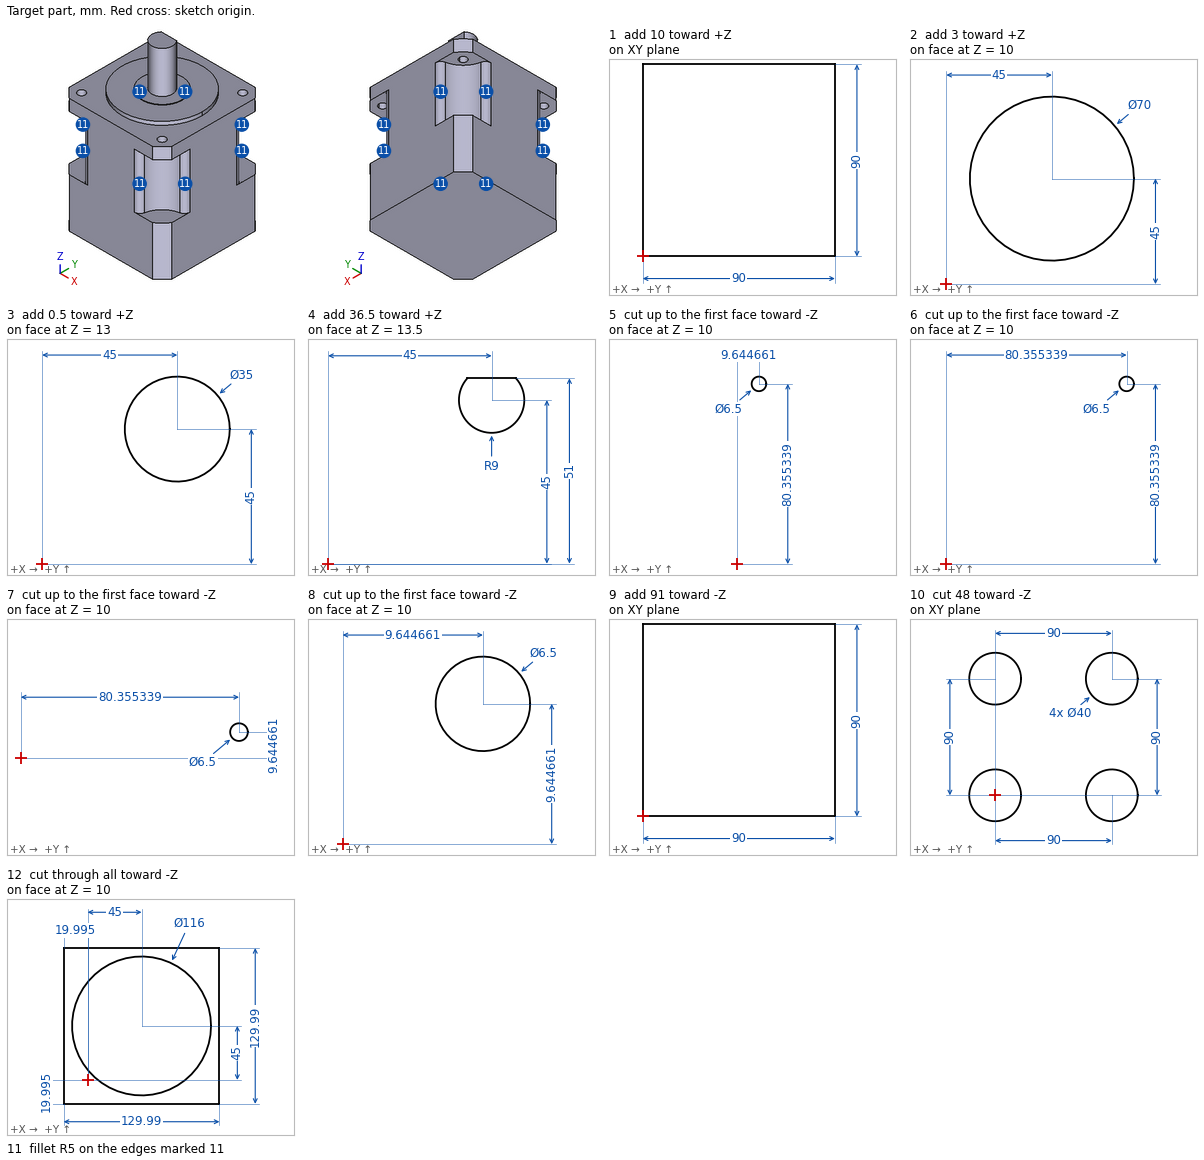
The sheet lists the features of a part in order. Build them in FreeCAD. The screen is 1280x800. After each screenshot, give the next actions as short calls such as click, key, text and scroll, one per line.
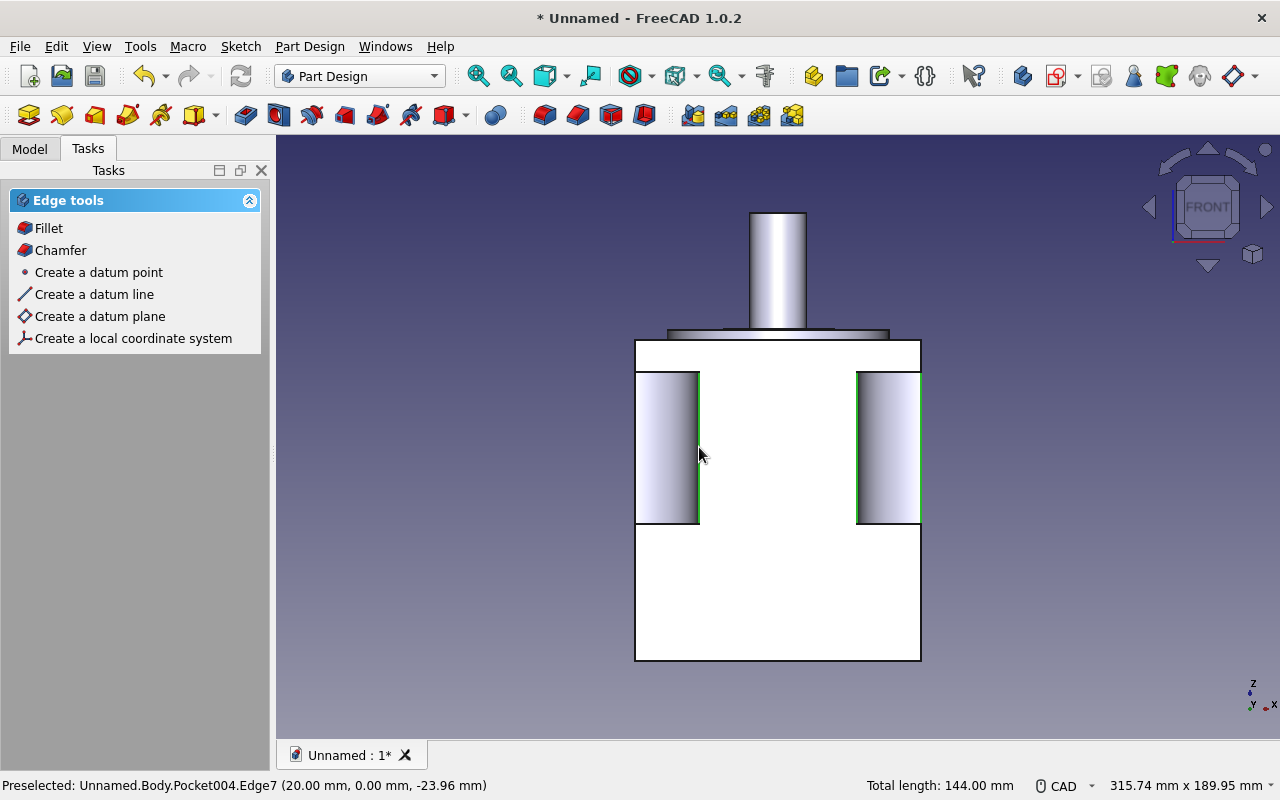
key(3)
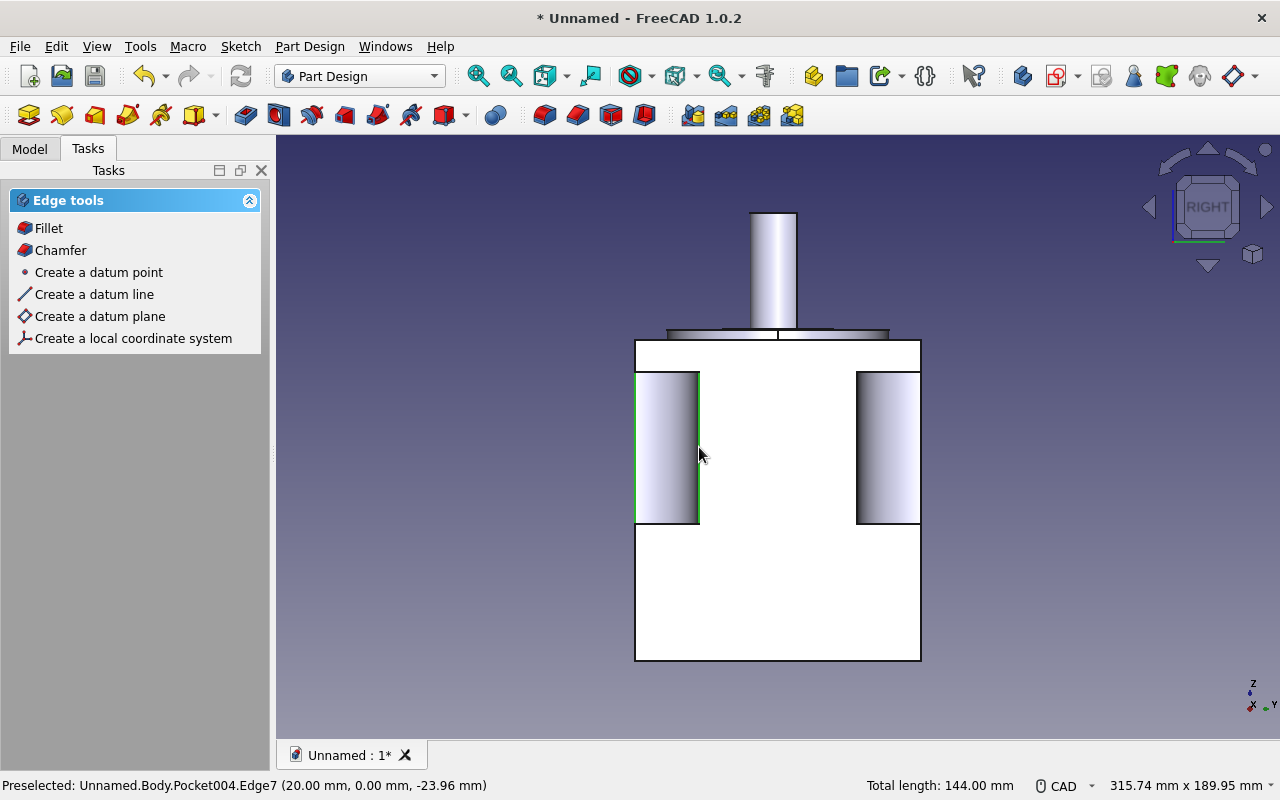
click(857, 447, ctrl)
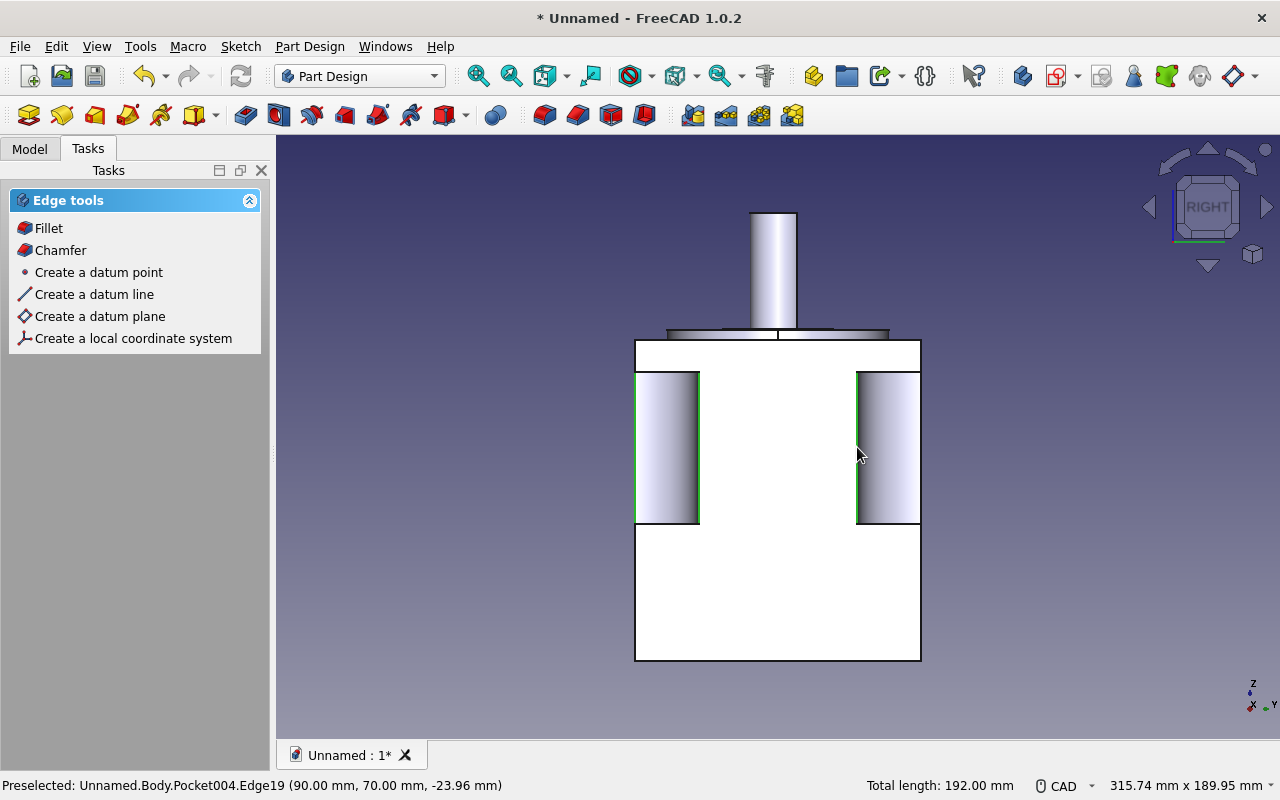
key(5)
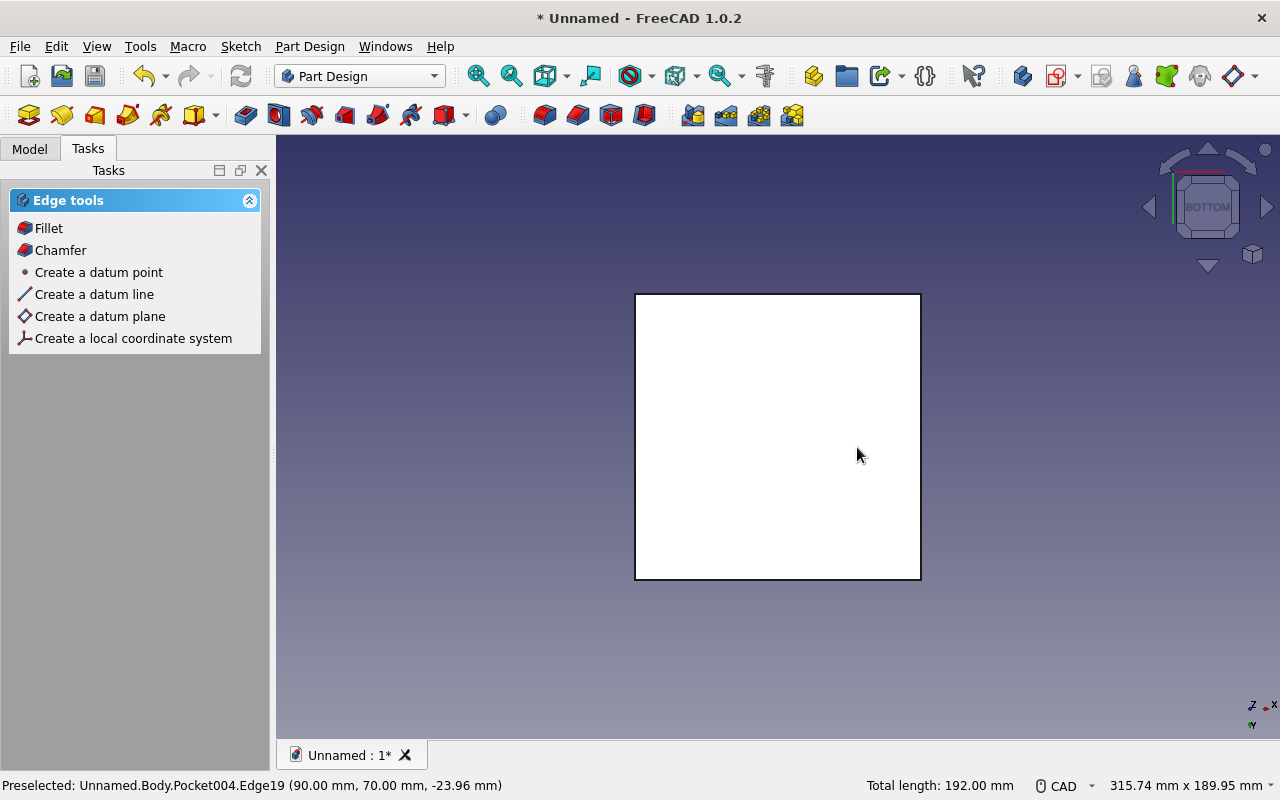
key(4)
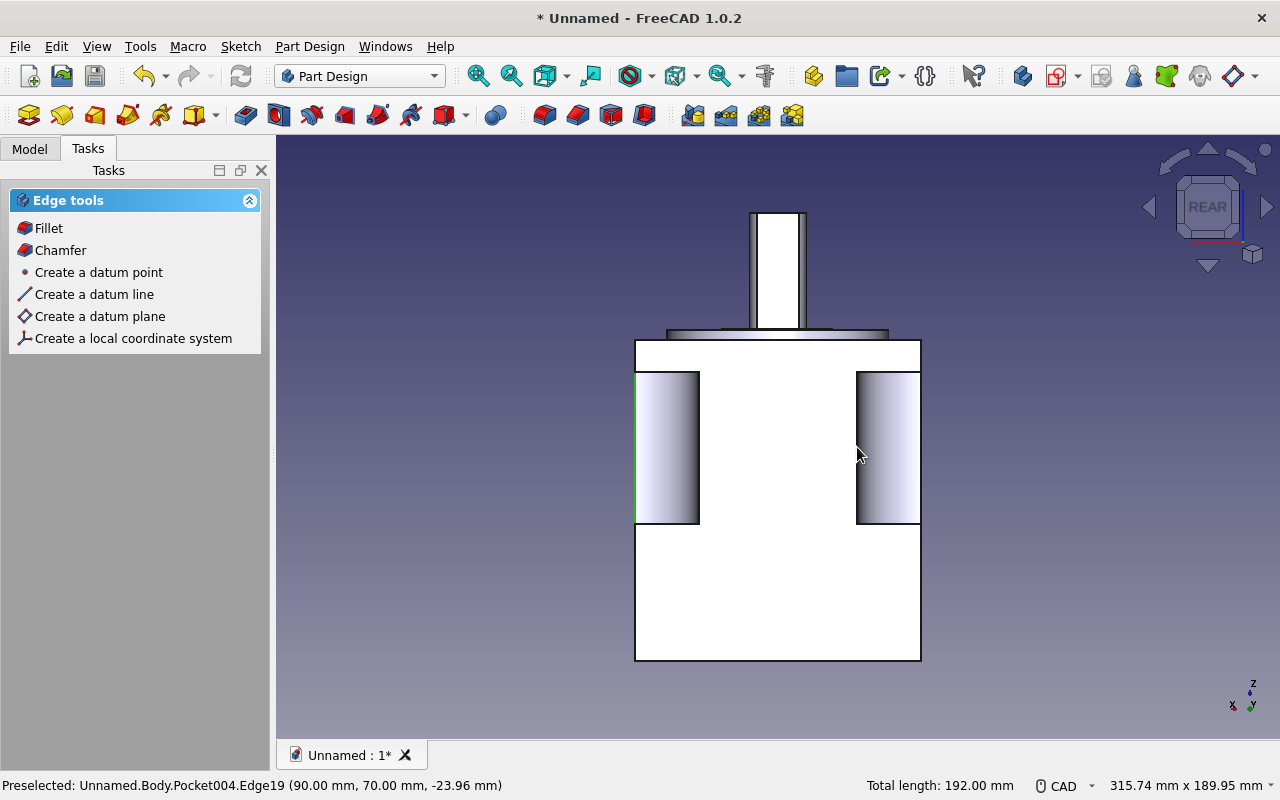
click(699, 447, ctrl)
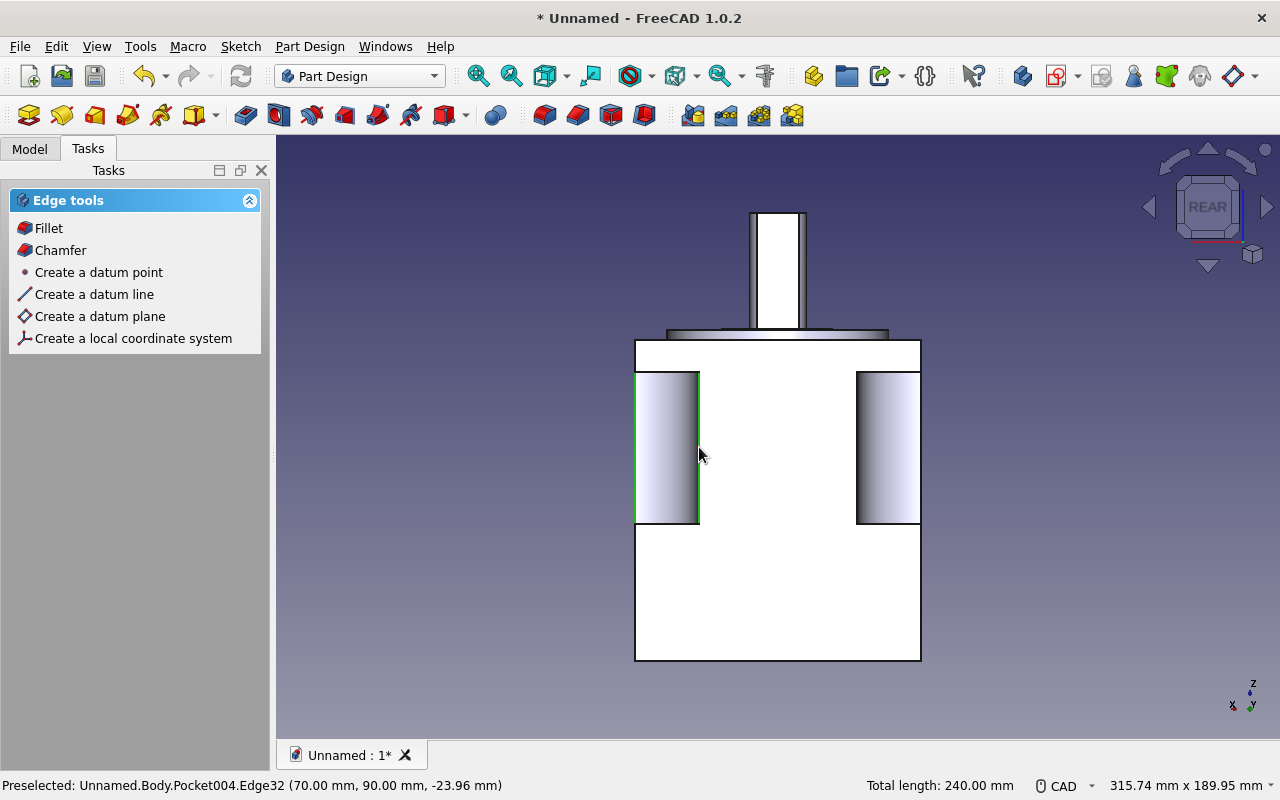
click(857, 447, ctrl)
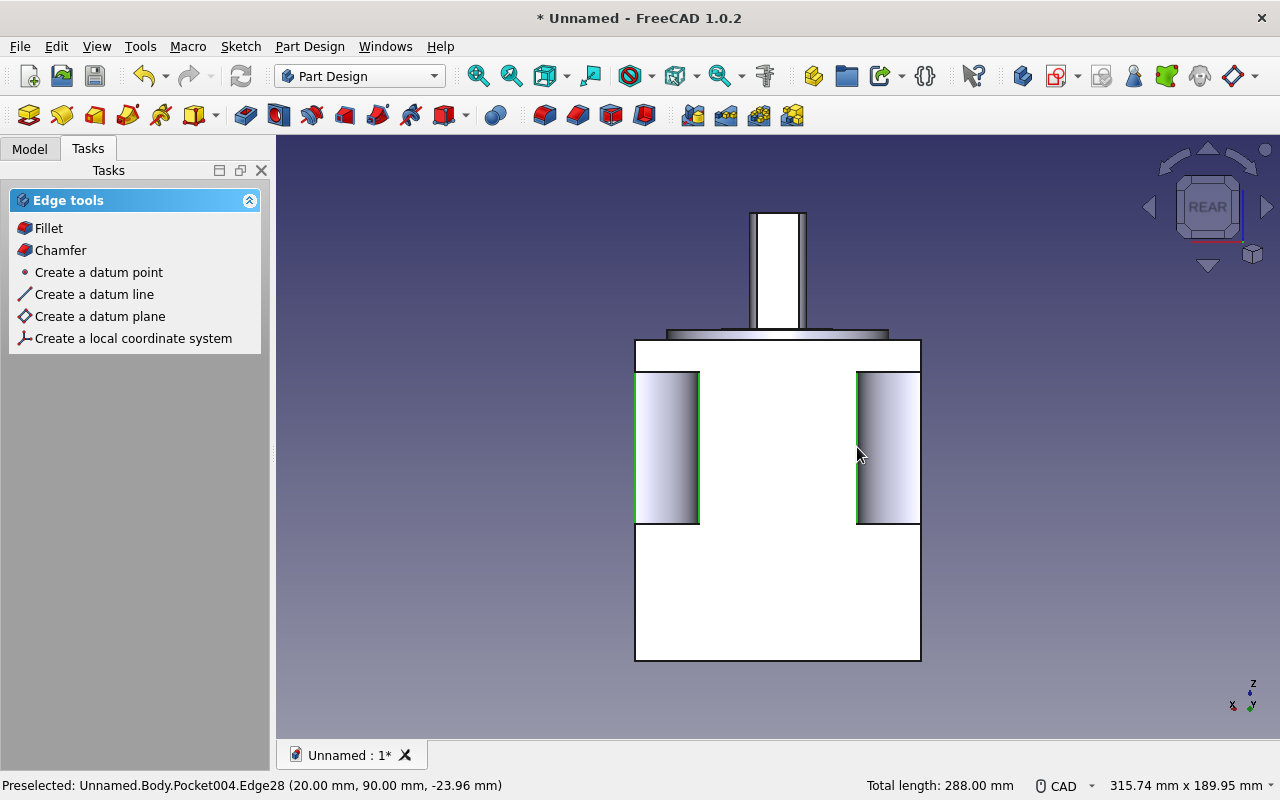
key(6)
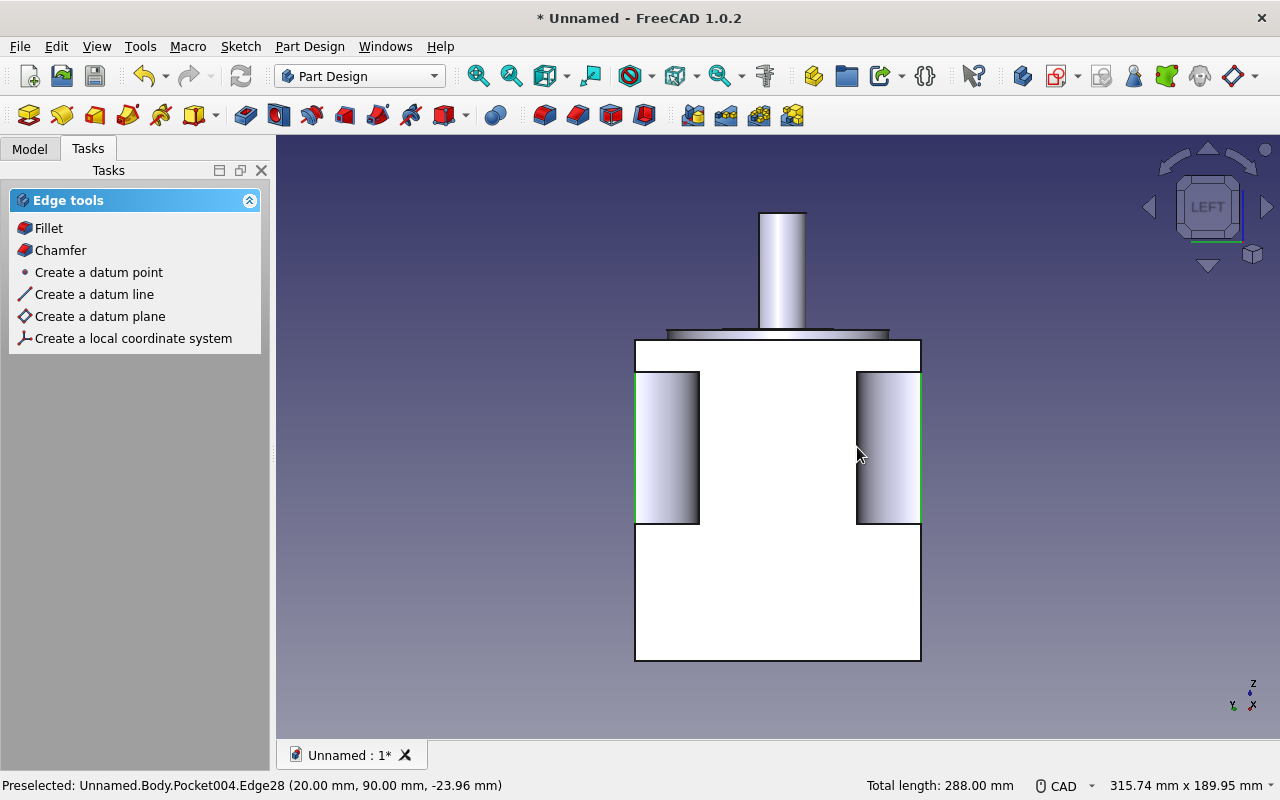
click(699, 447, ctrl)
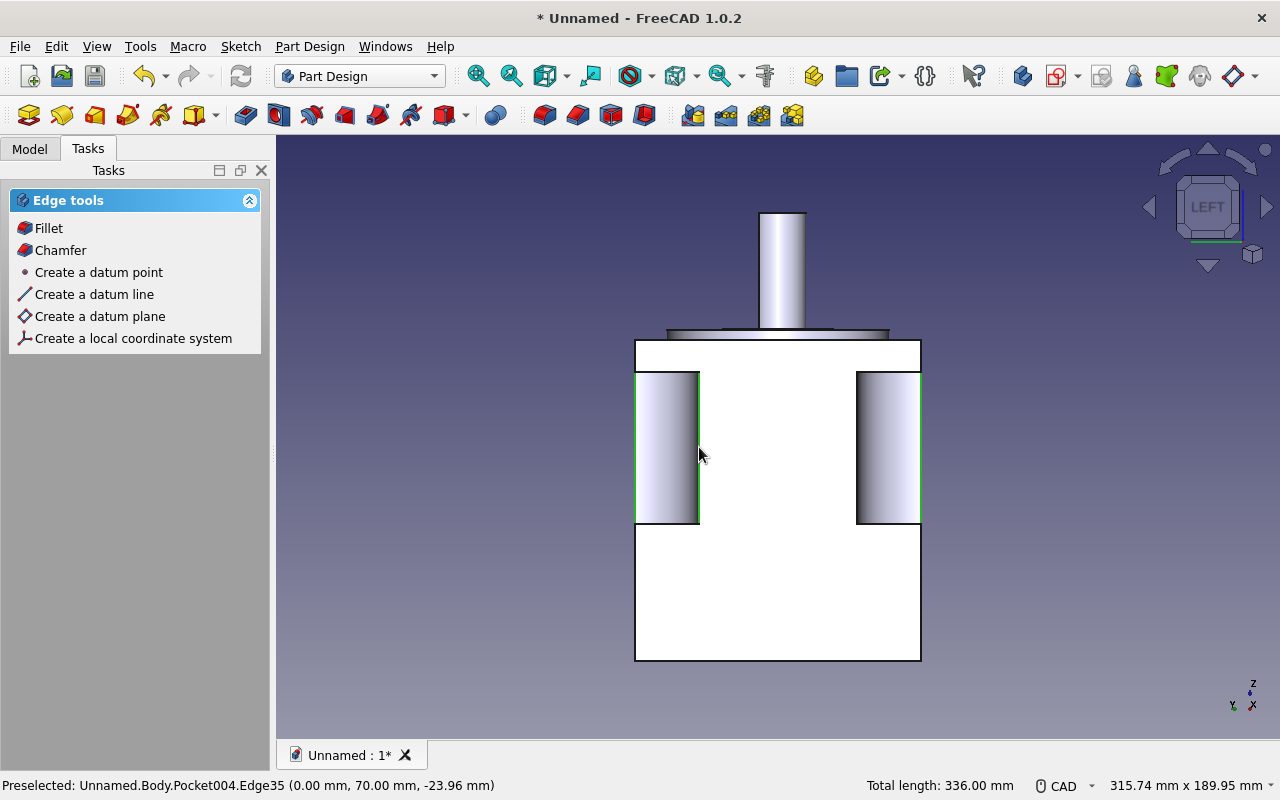
key(v)
key(3)